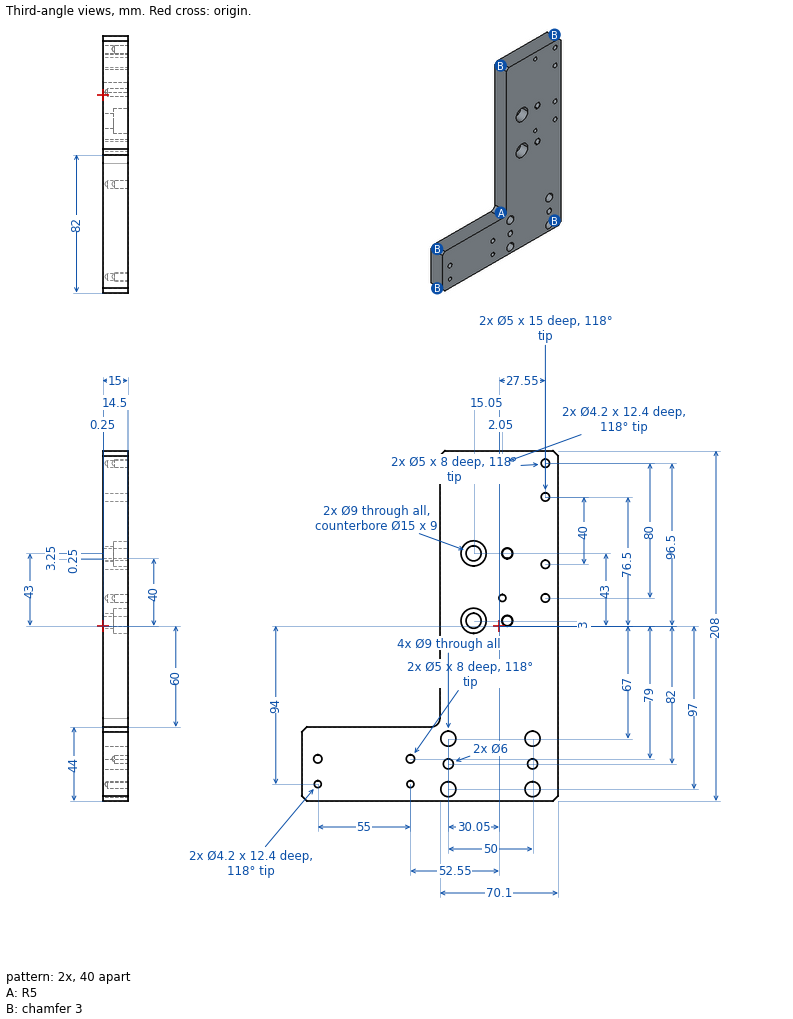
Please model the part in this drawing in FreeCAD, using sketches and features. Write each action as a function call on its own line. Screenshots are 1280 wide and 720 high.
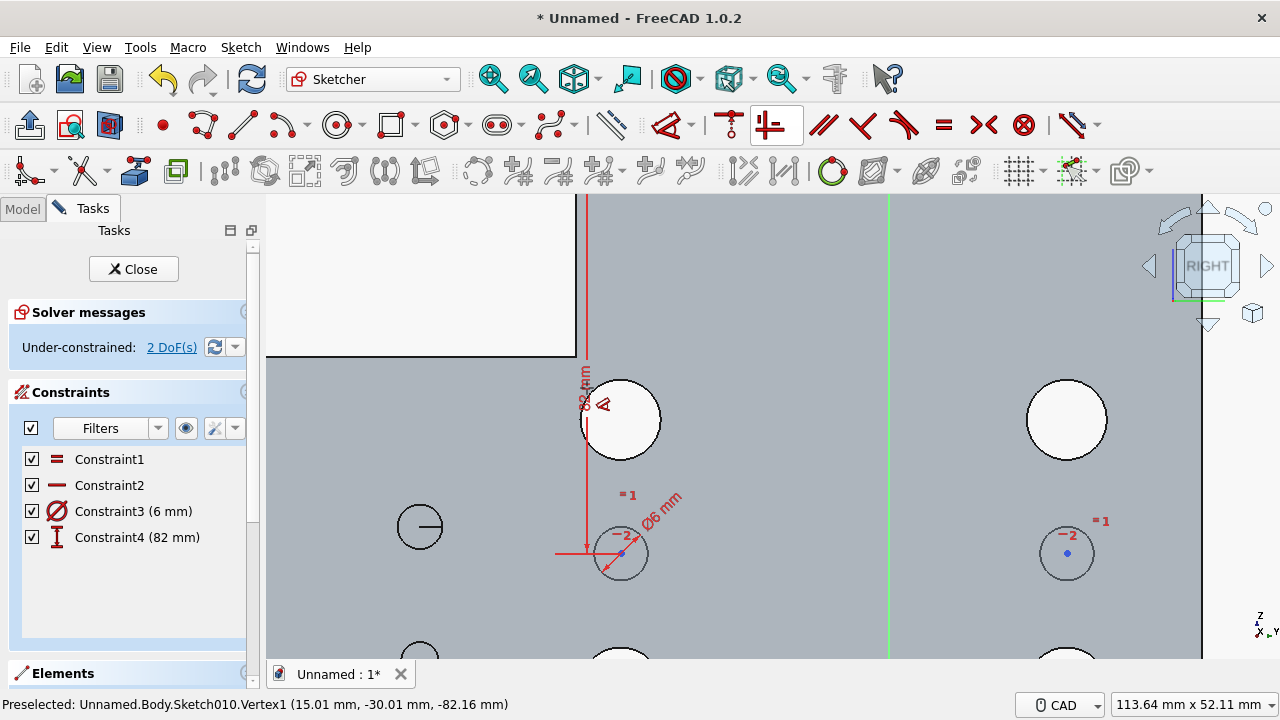
click(621, 554)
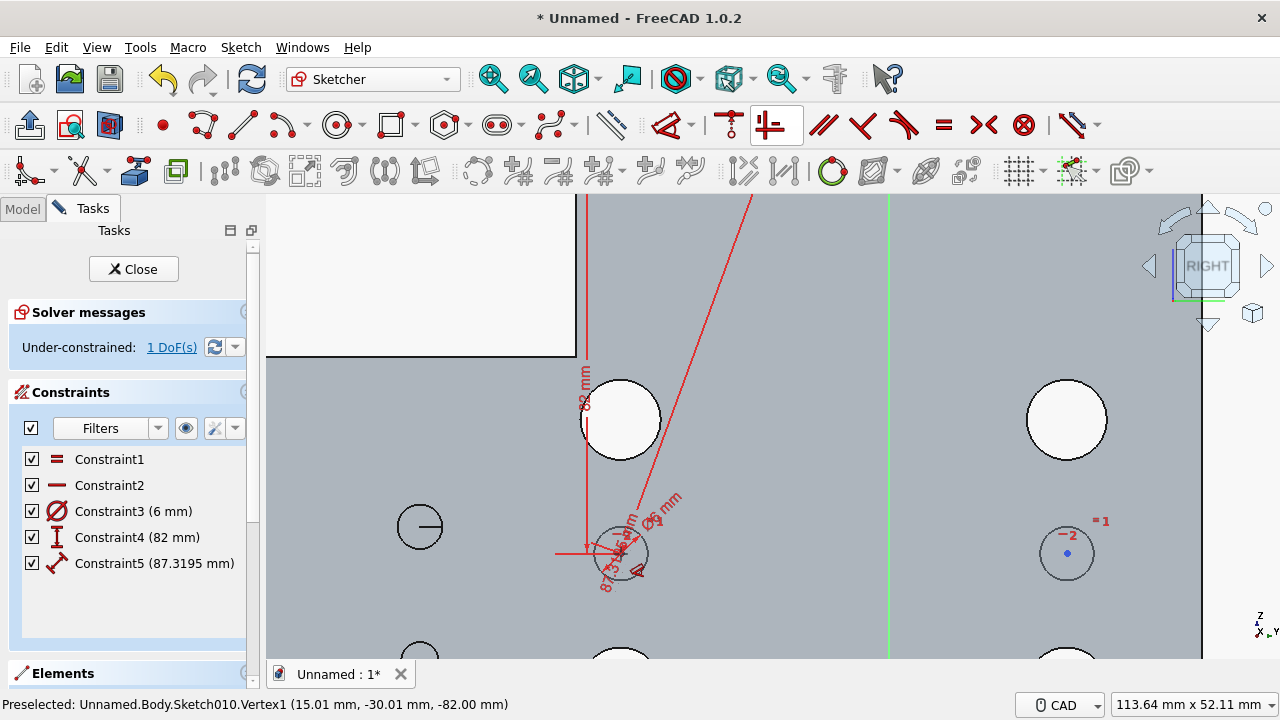
click(1067, 554)
click(844, 588)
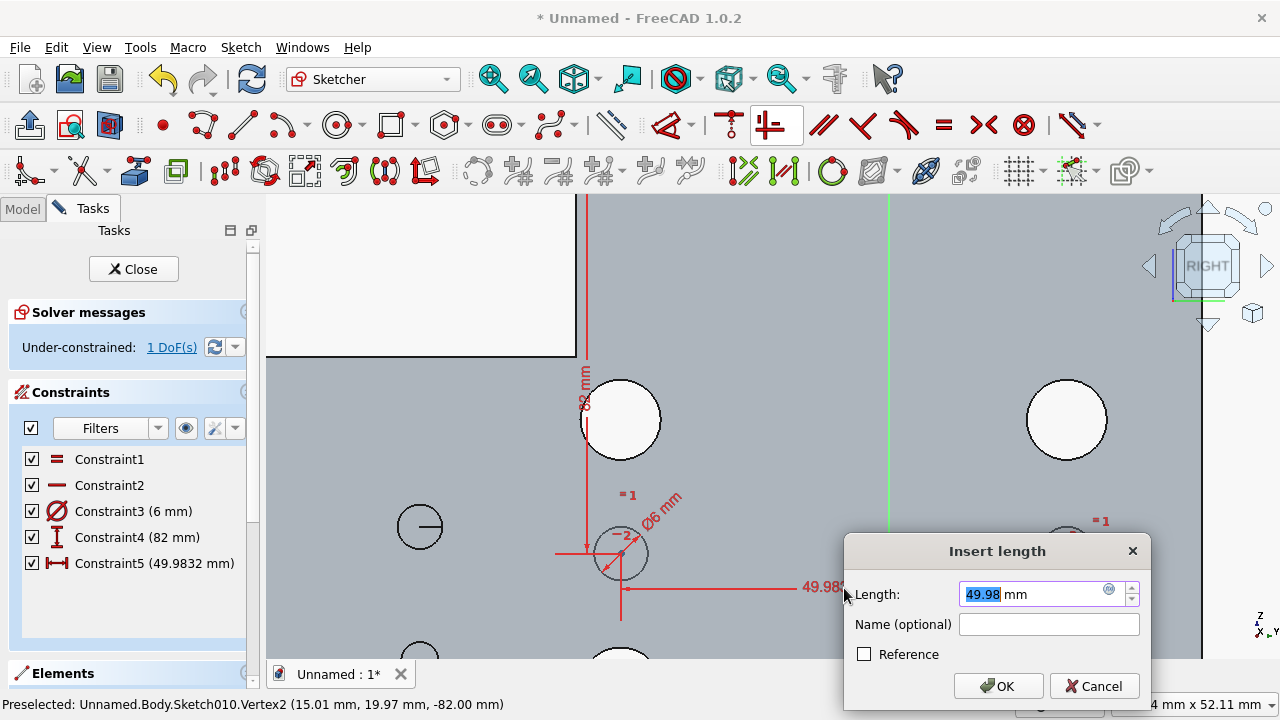
text(50)
key(Return)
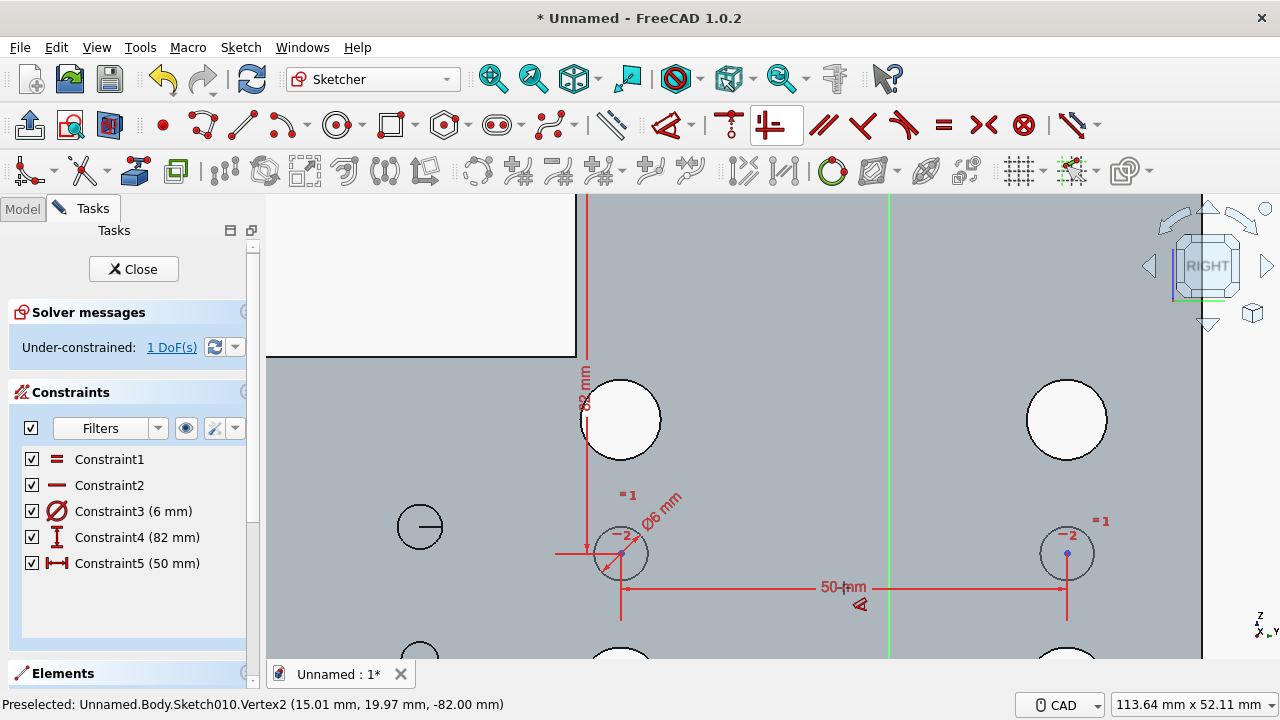
click(621, 554)
click(755, 588)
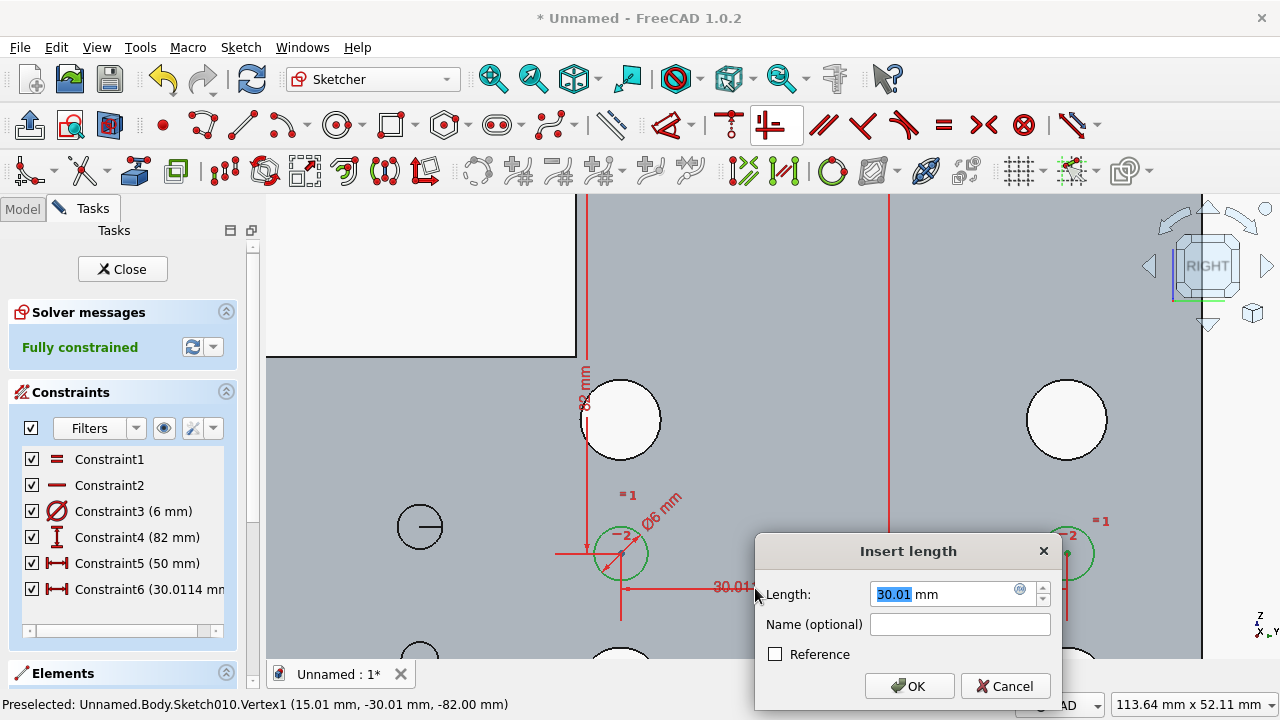
text(30.05)
key(Return)
key(Escape)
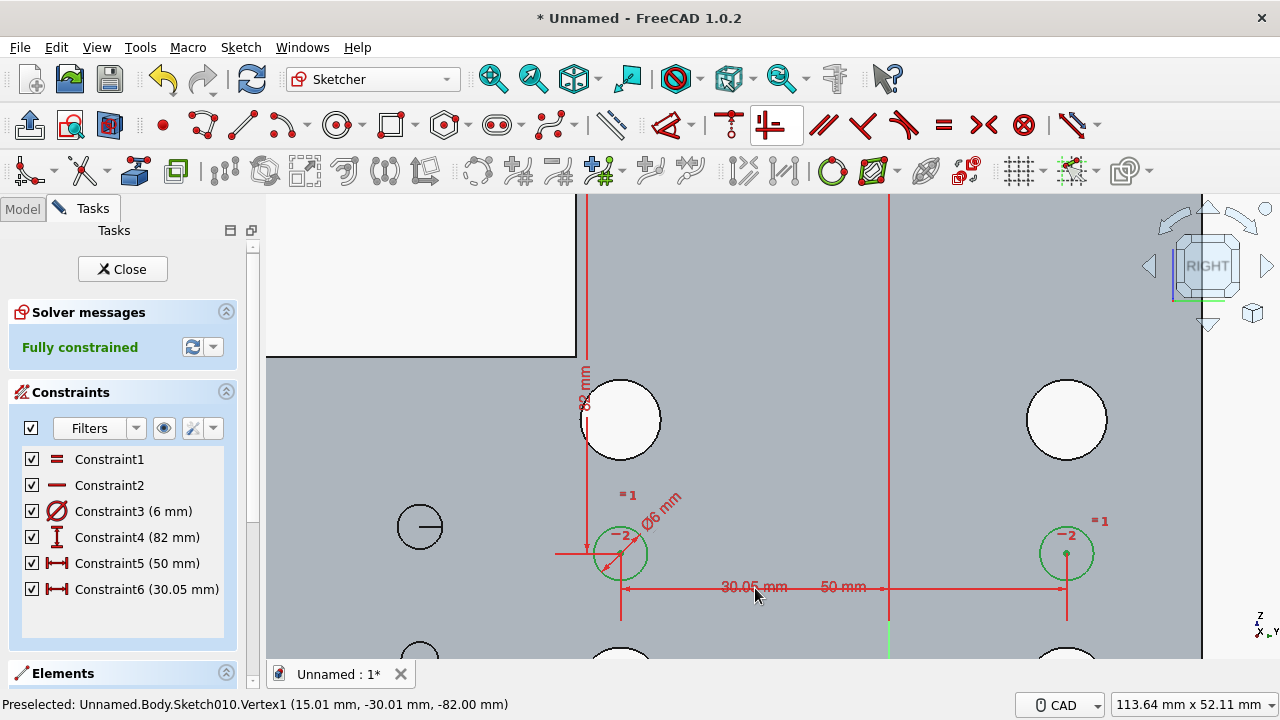
click(123, 269)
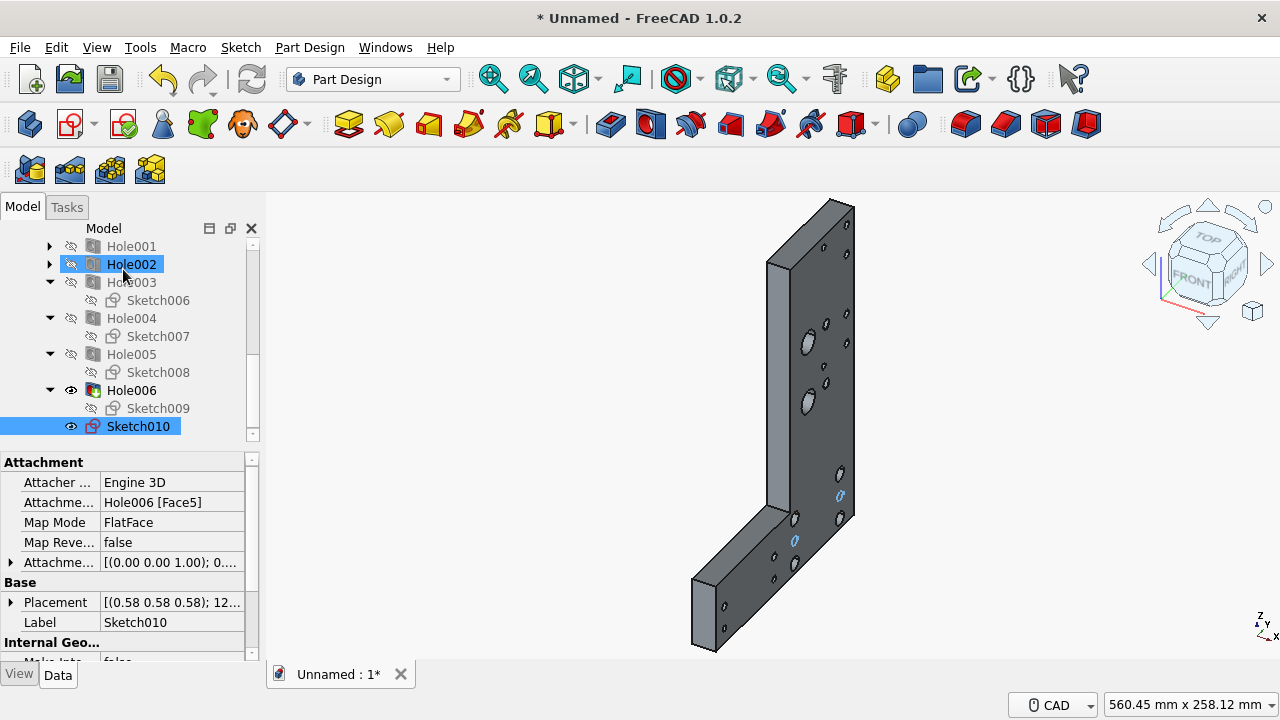
click(612, 124)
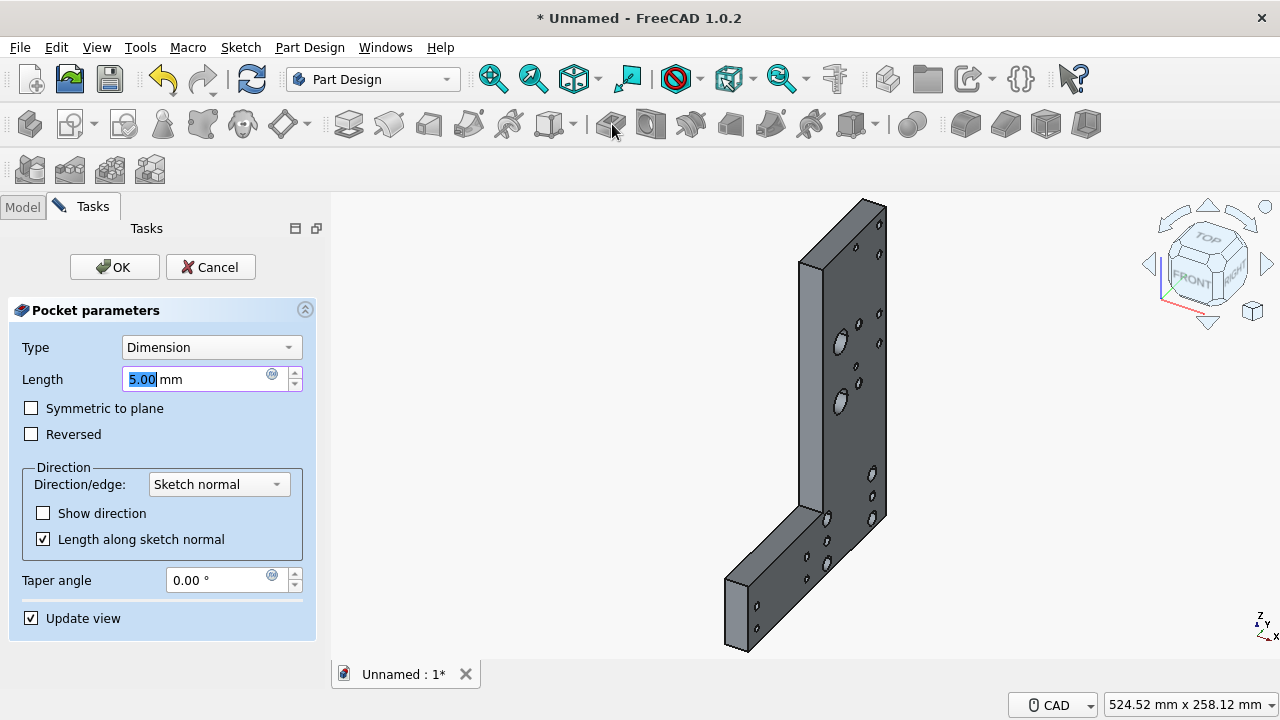
click(212, 348)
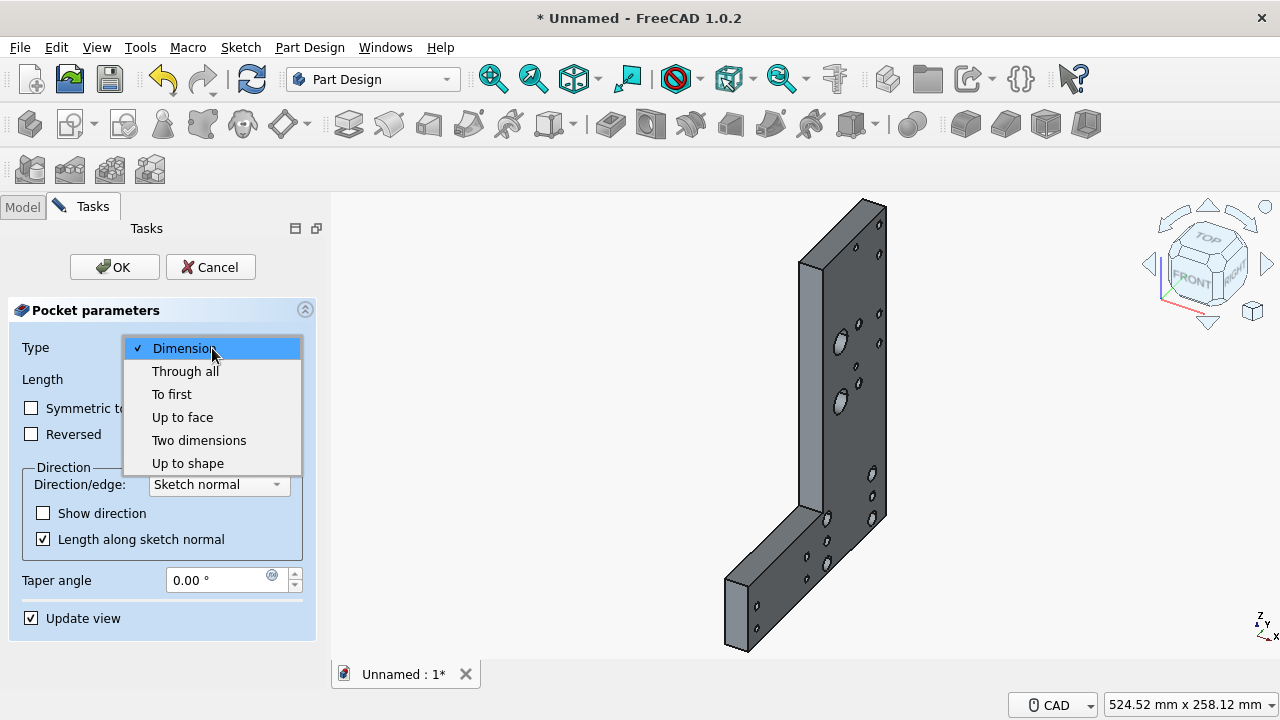
click(212, 372)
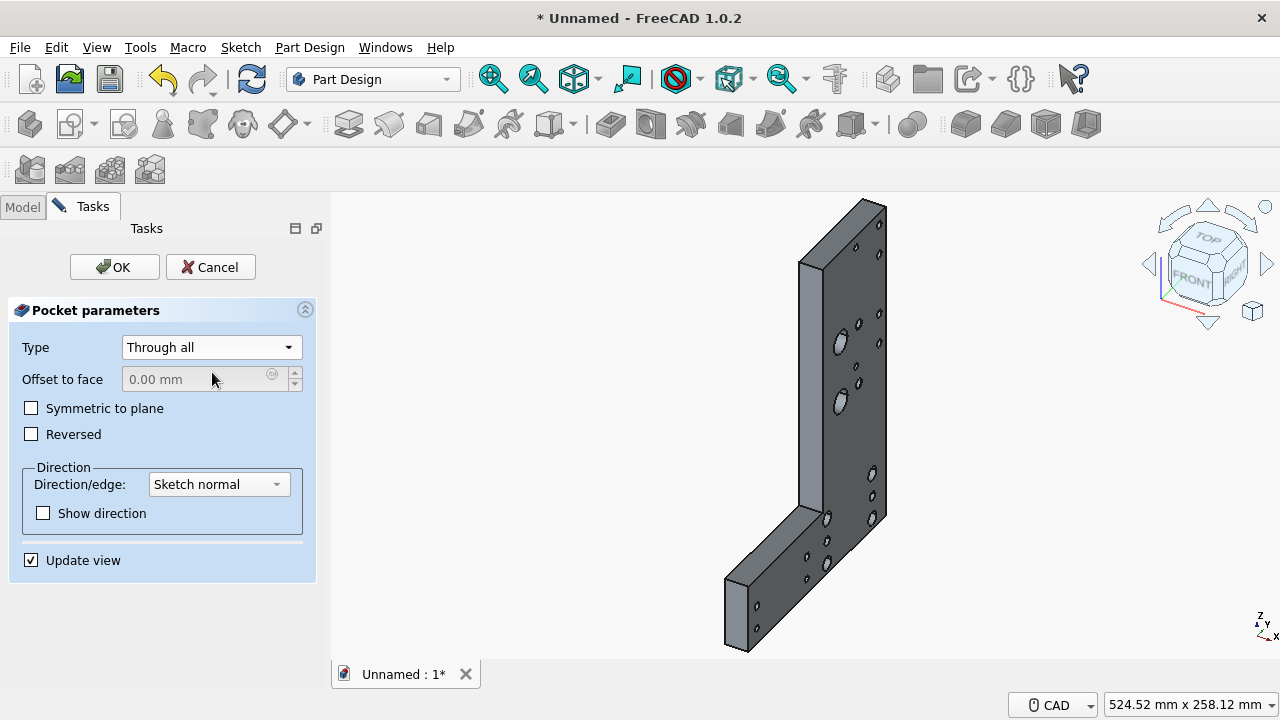
click(115, 267)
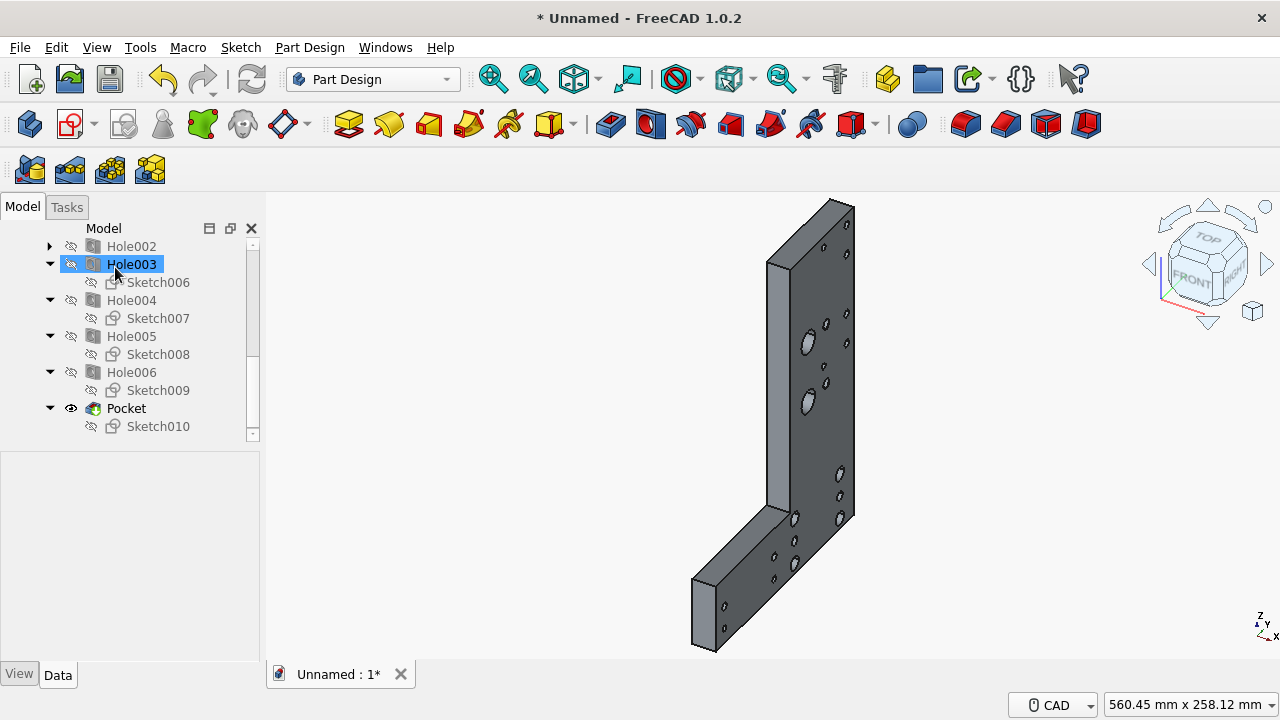
key(0)